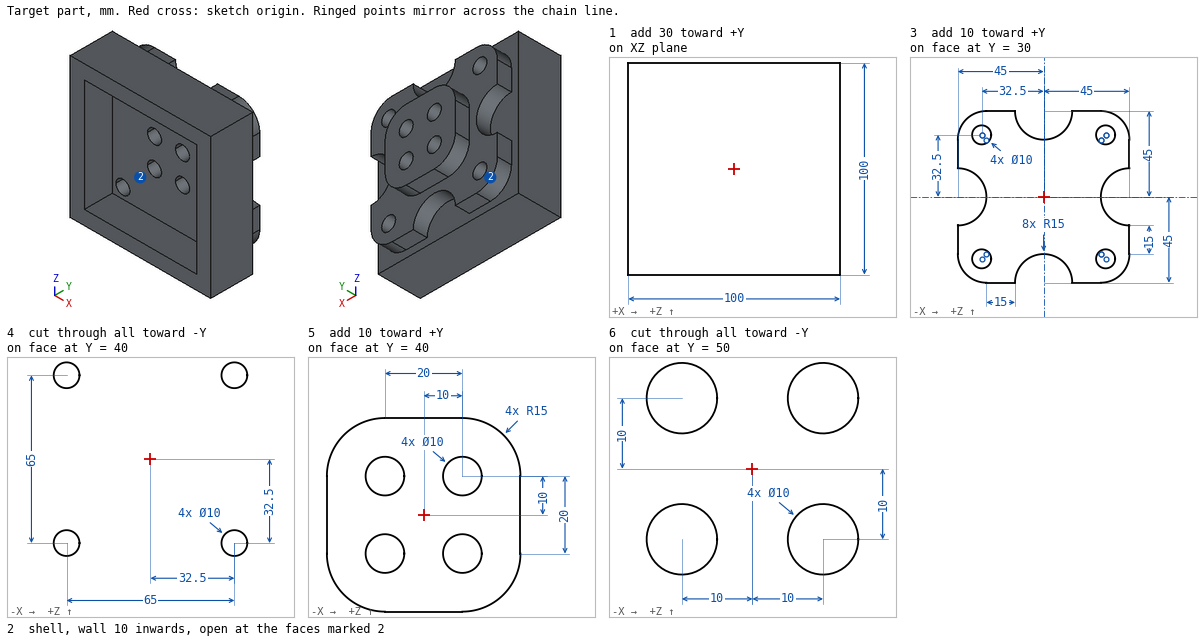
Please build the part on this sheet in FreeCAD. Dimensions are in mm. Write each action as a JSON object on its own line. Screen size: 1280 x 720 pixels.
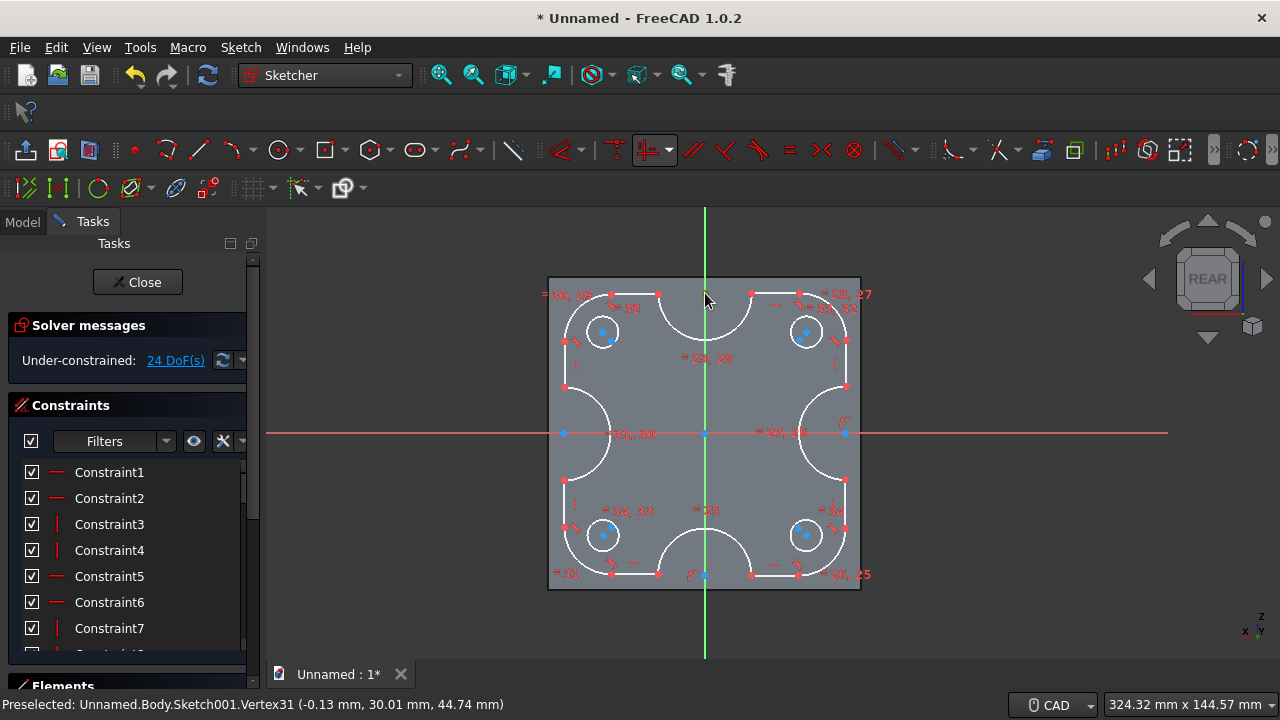
{"action": "left_click", "coordinate": [705, 603]}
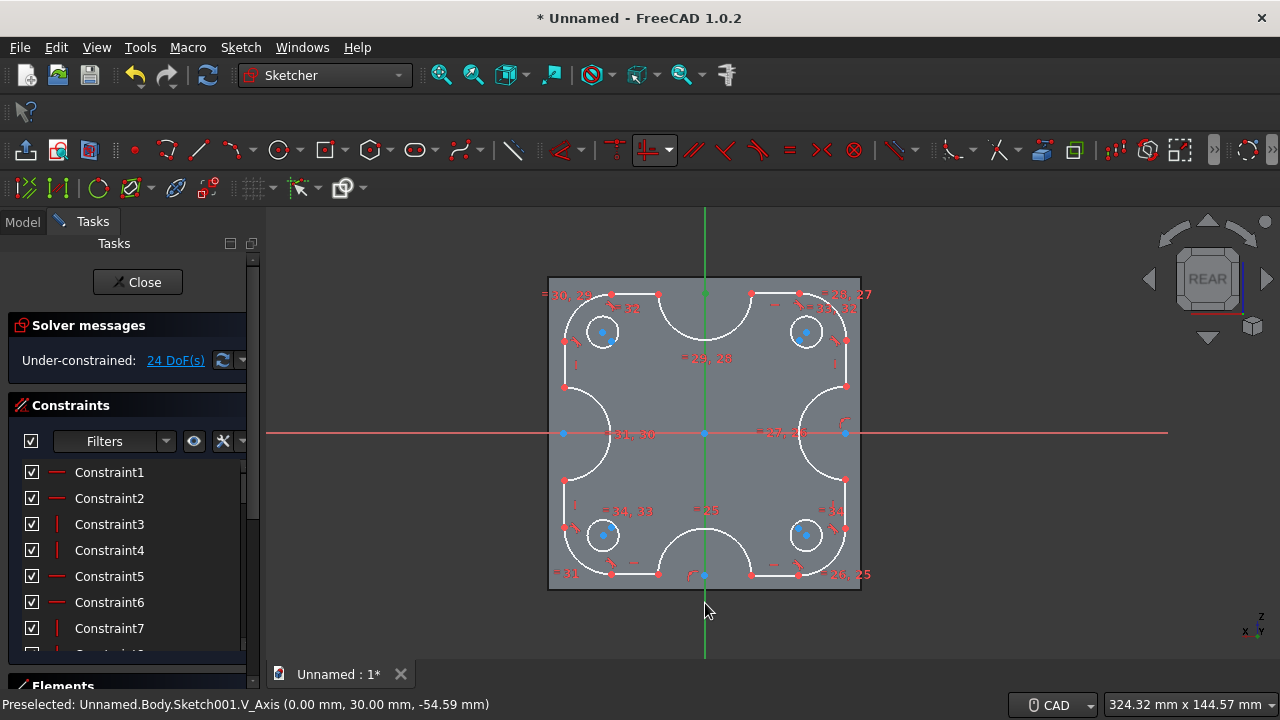
{"action": "left_click", "coordinate": [616, 150]}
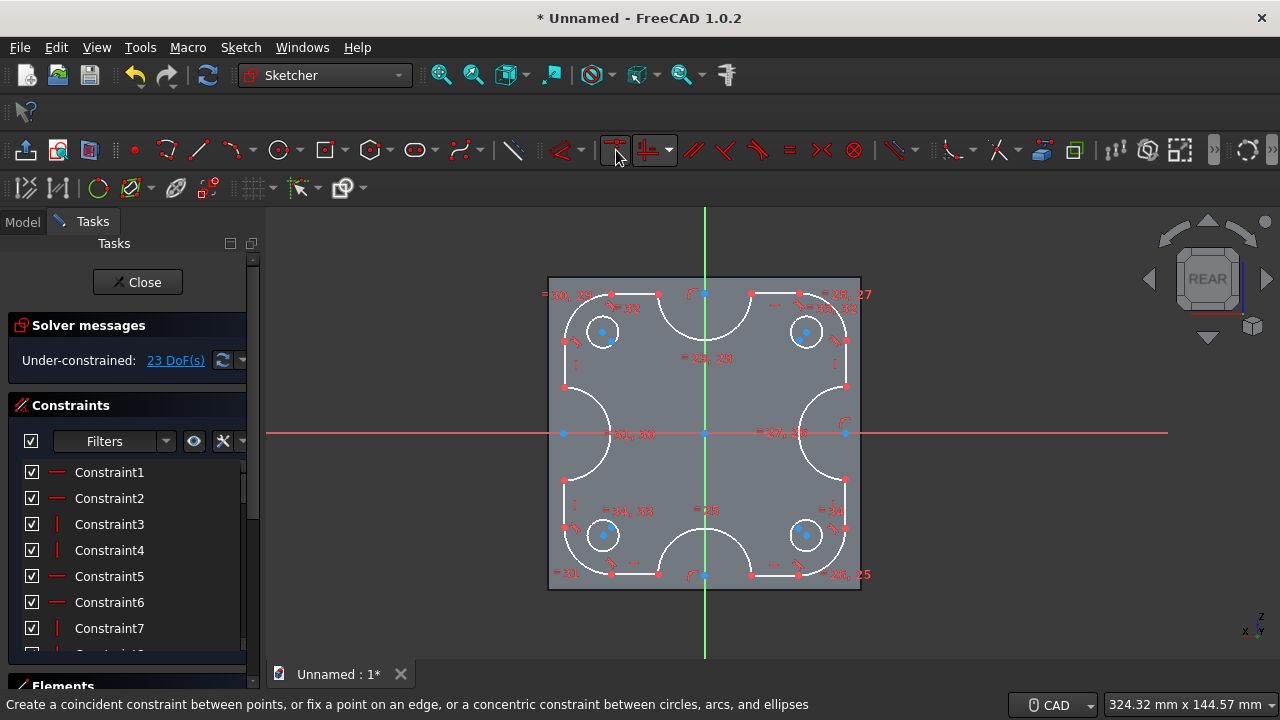
{"action": "left_click", "coordinate": [564, 434]}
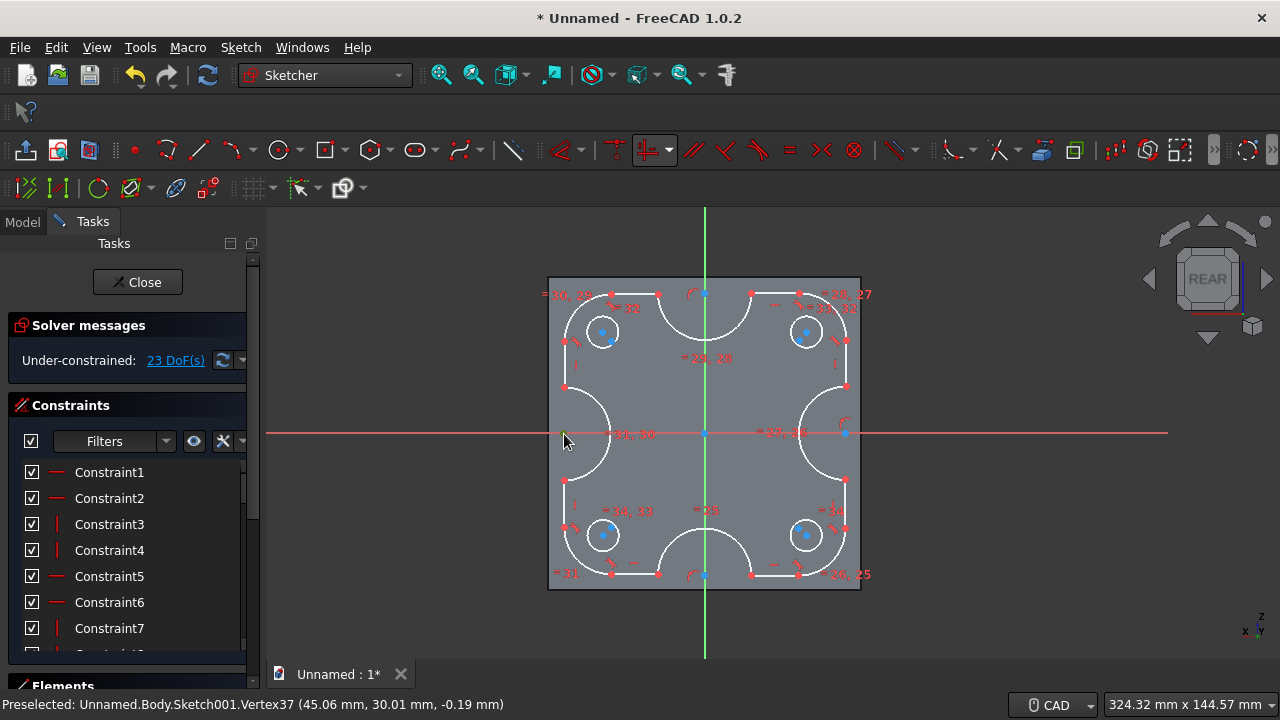
{"action": "left_click", "coordinate": [353, 433]}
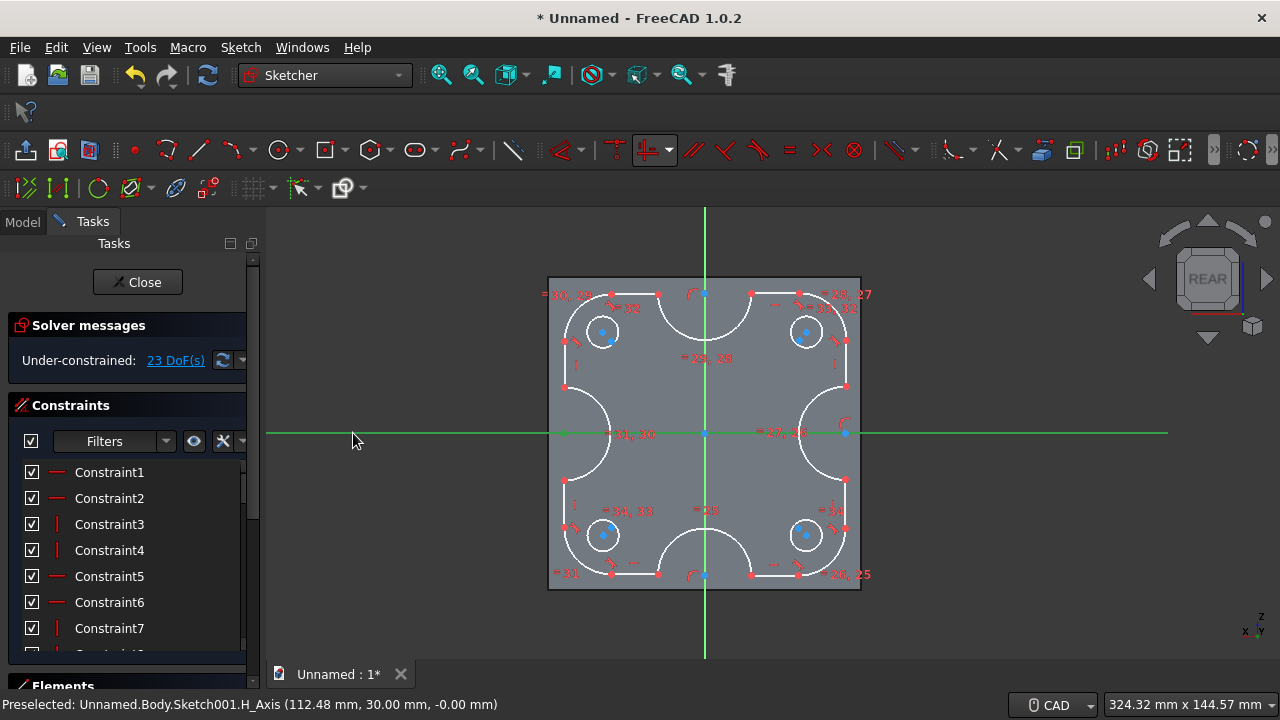
{"action": "left_click", "coordinate": [616, 150]}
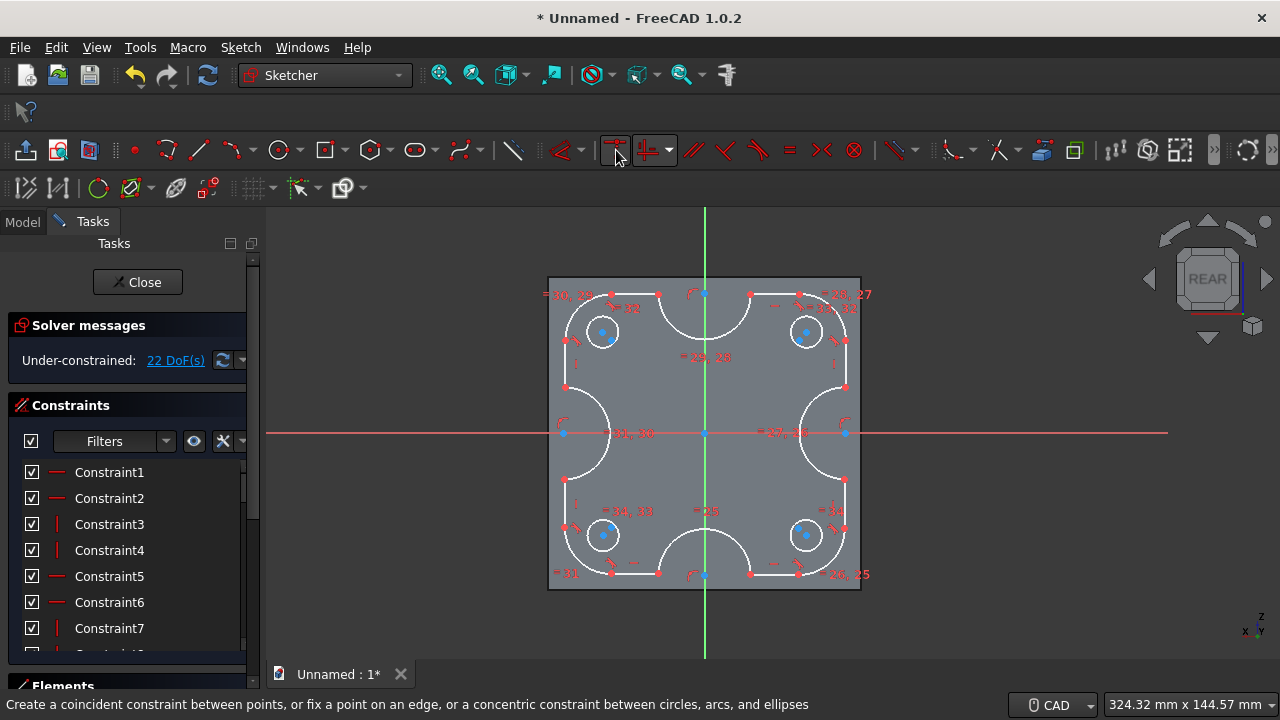
{"action": "left_click", "coordinate": [799, 529]}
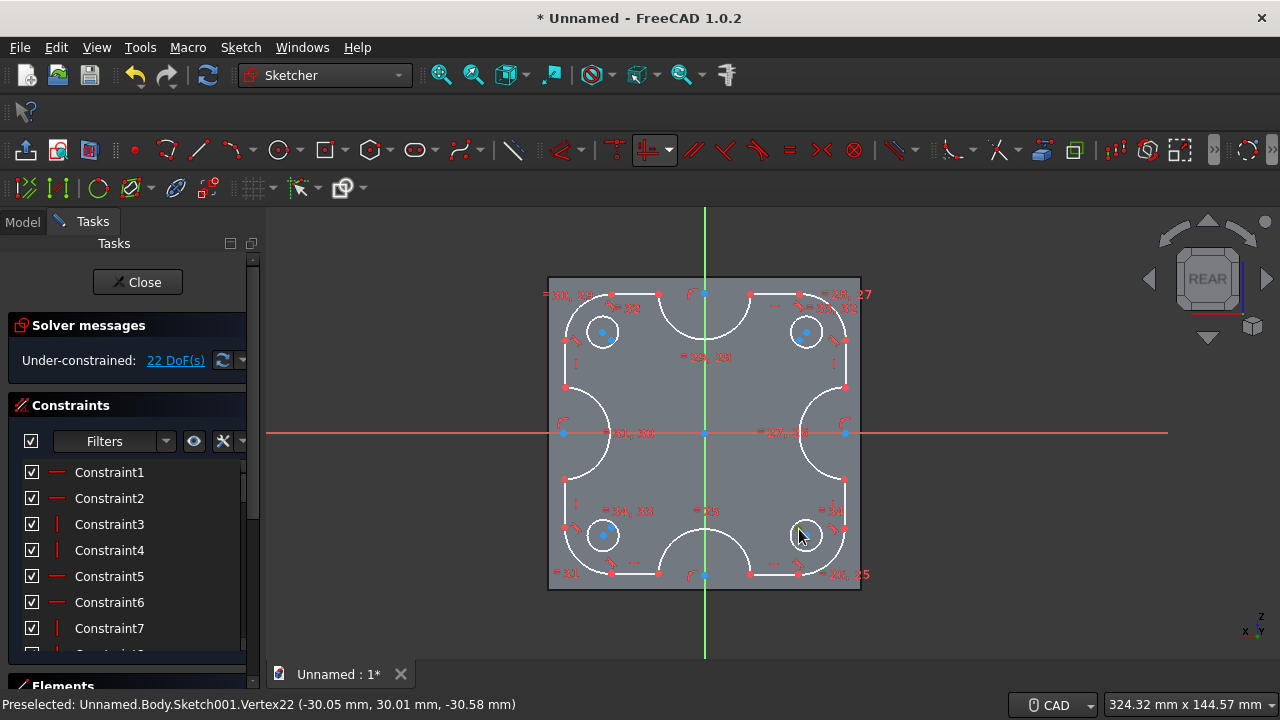
{"action": "left_click", "coordinate": [800, 340]}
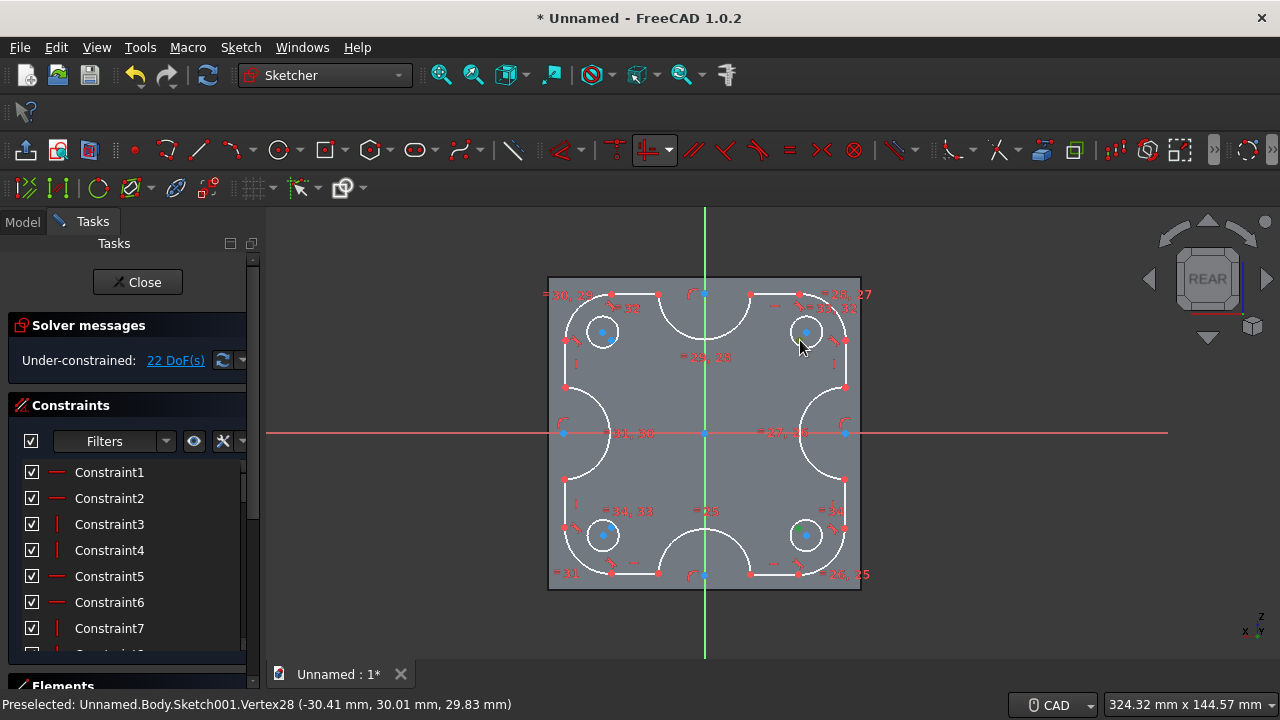
{"action": "left_click", "coordinate": [353, 433]}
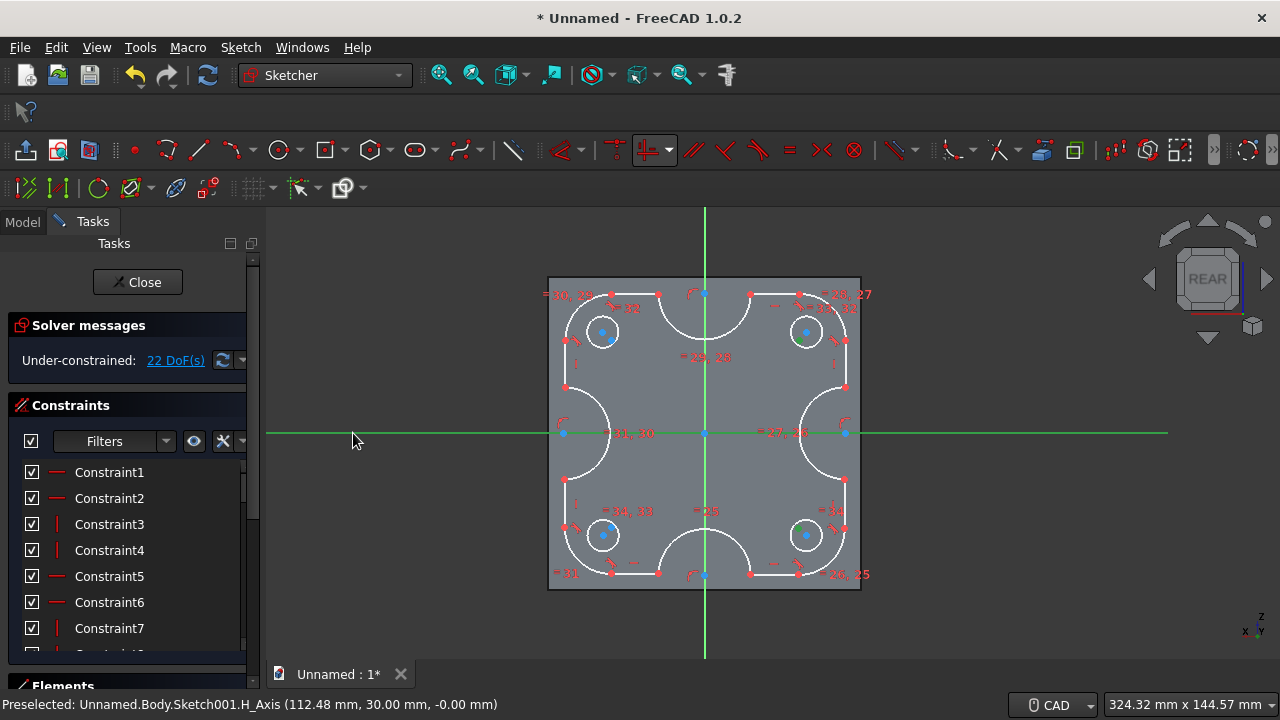
{"action": "left_click", "coordinate": [822, 150]}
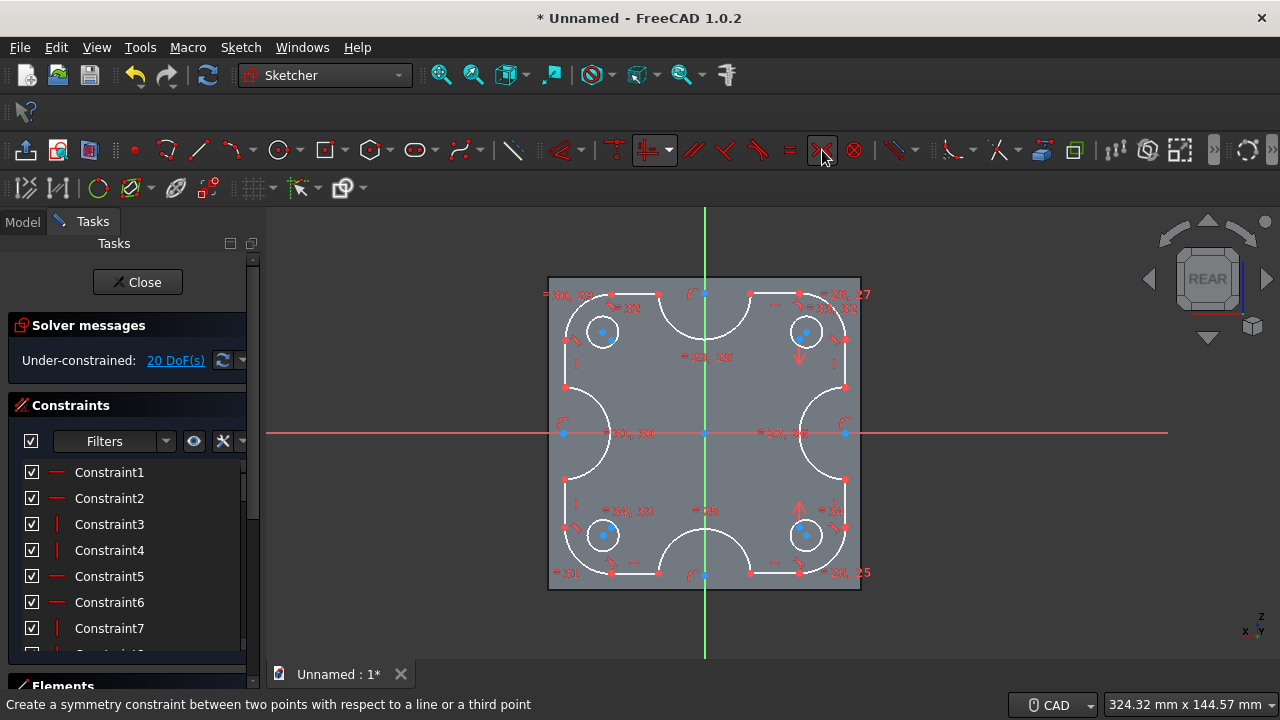
{"action": "left_click", "coordinate": [799, 339]}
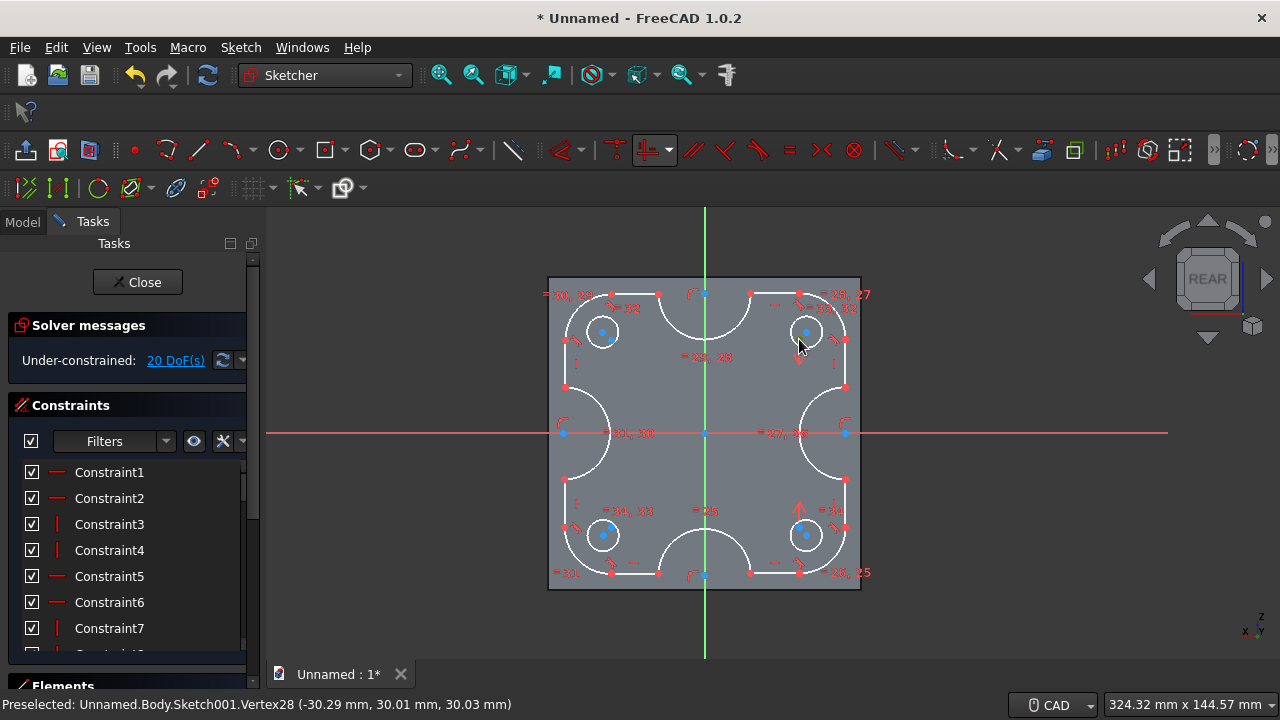
{"action": "left_click", "coordinate": [612, 341]}